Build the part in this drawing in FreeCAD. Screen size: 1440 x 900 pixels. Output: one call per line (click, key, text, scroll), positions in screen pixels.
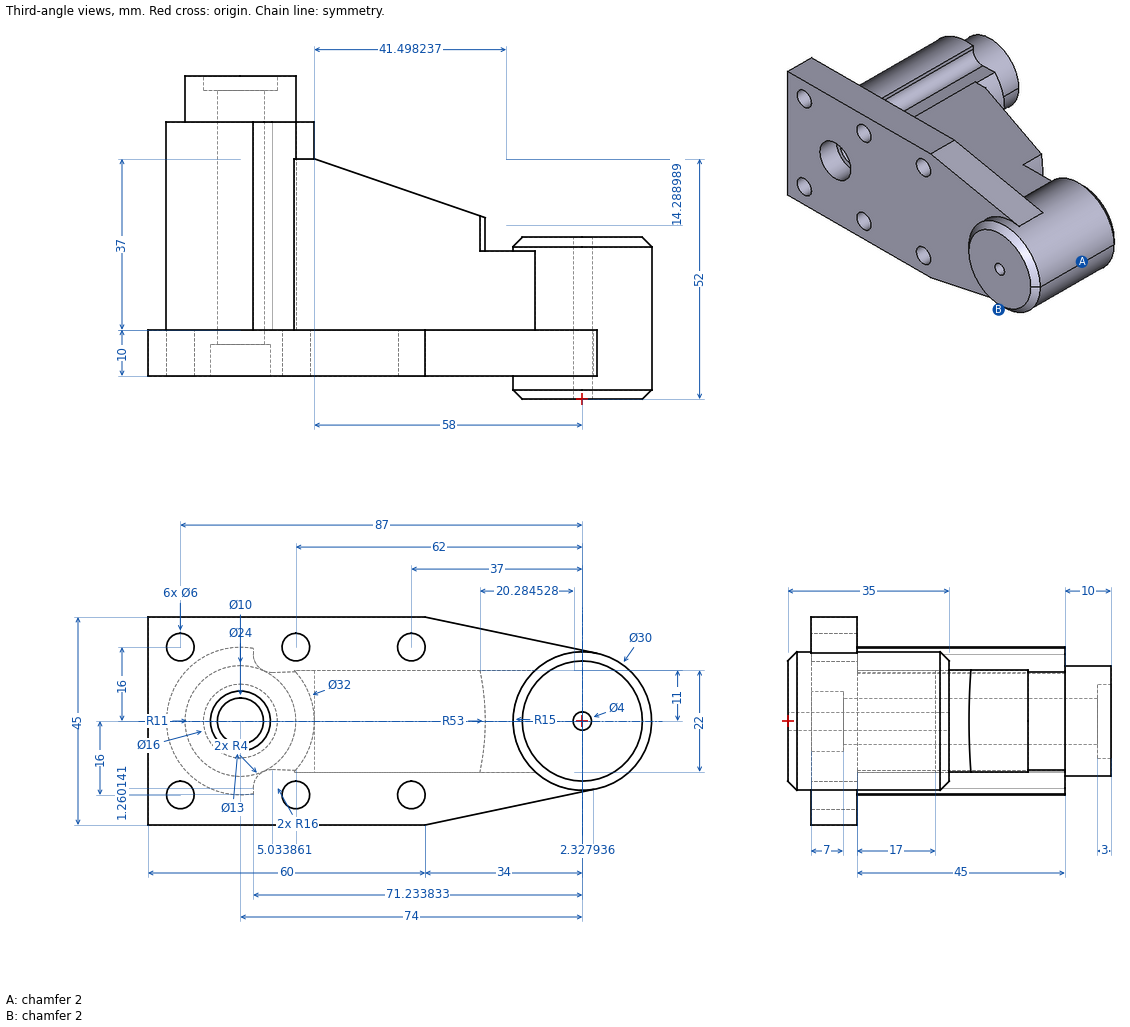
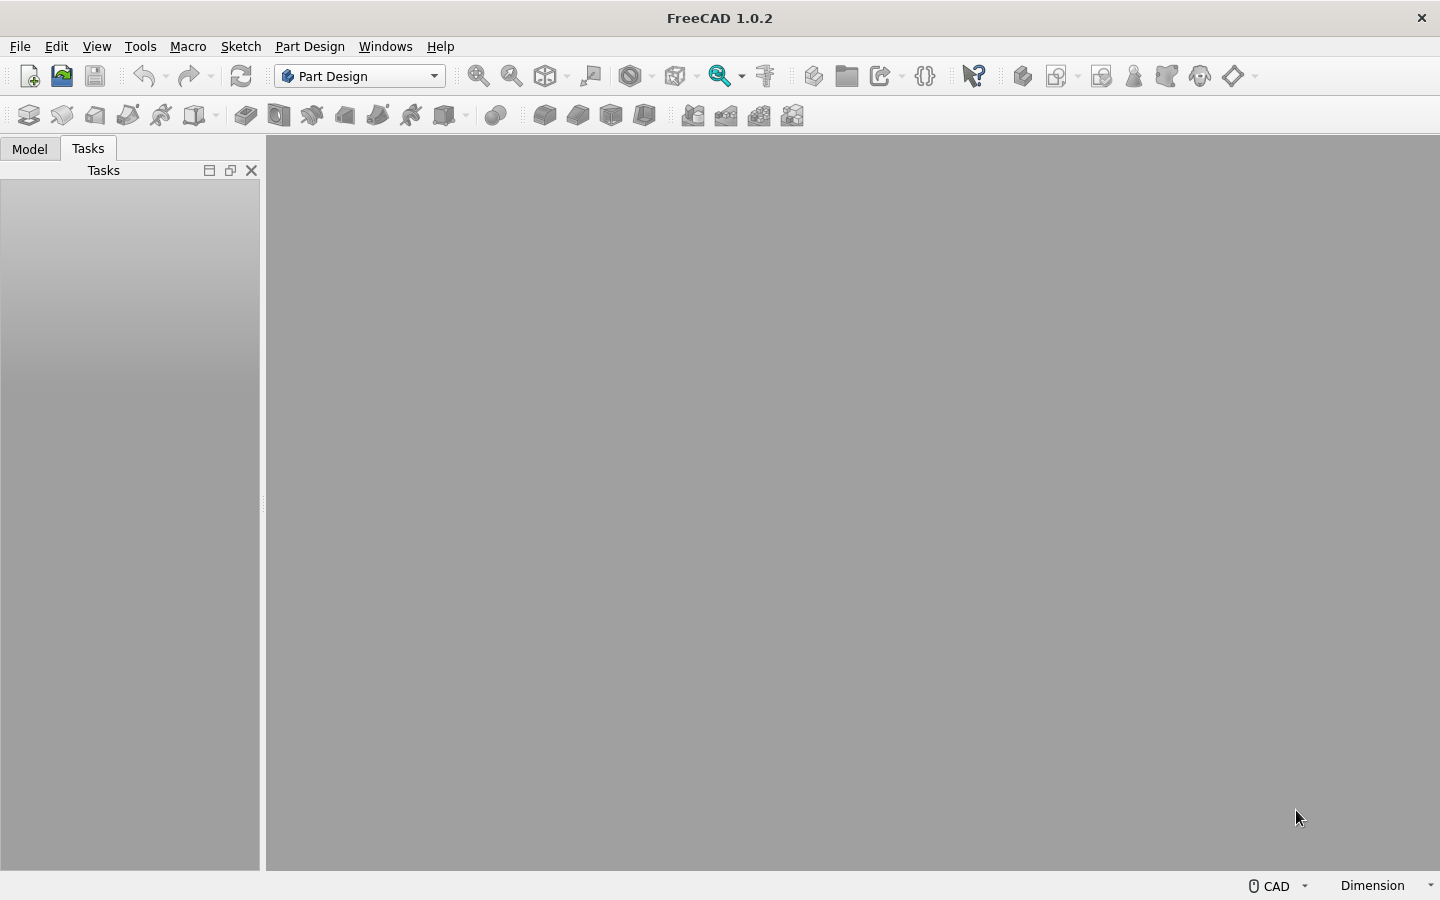
click(29, 76)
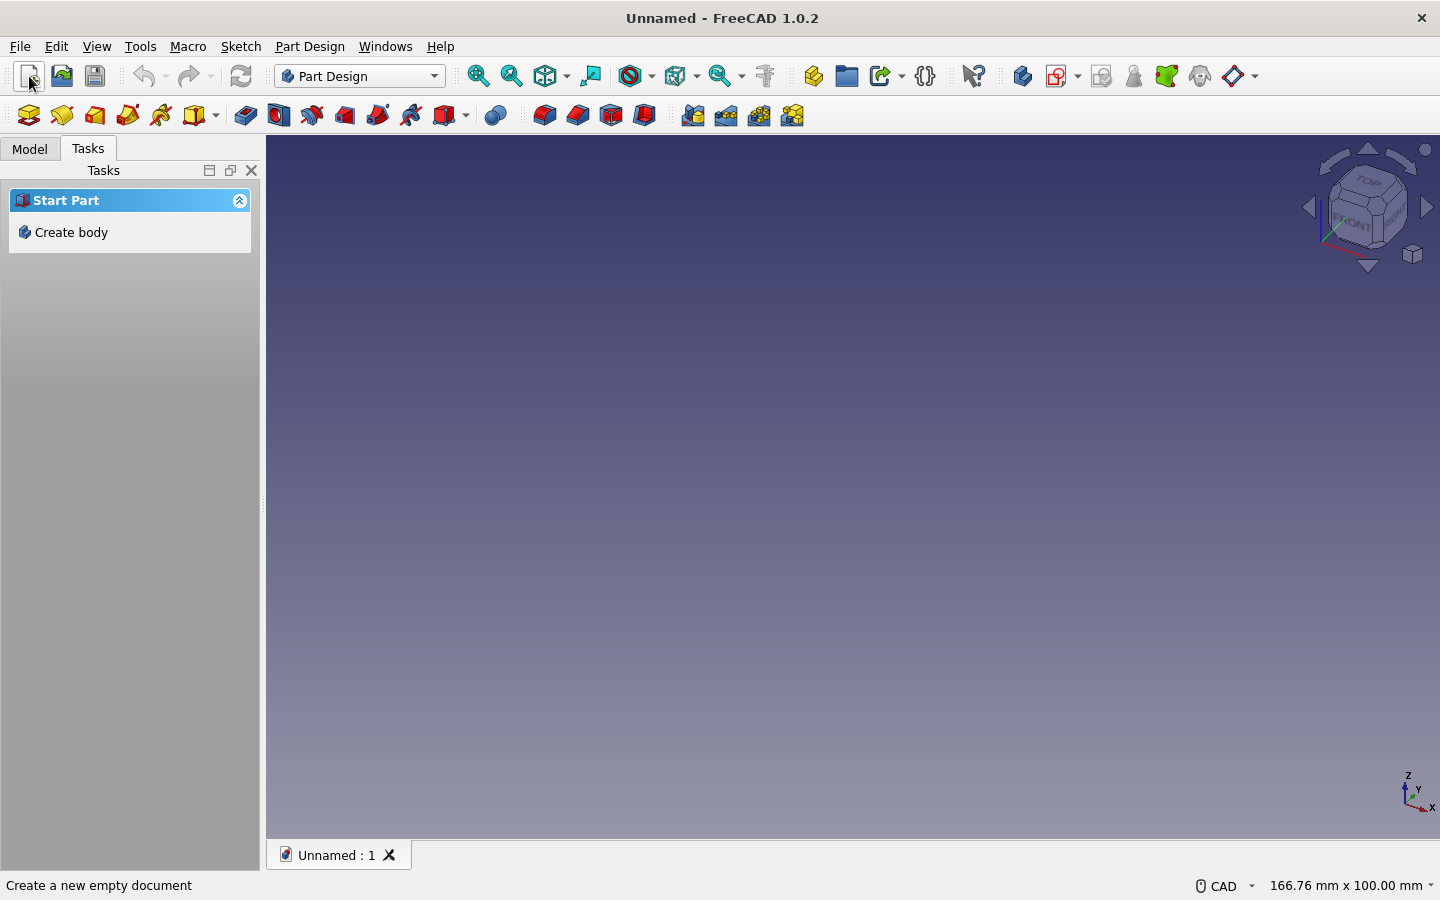
click(1056, 76)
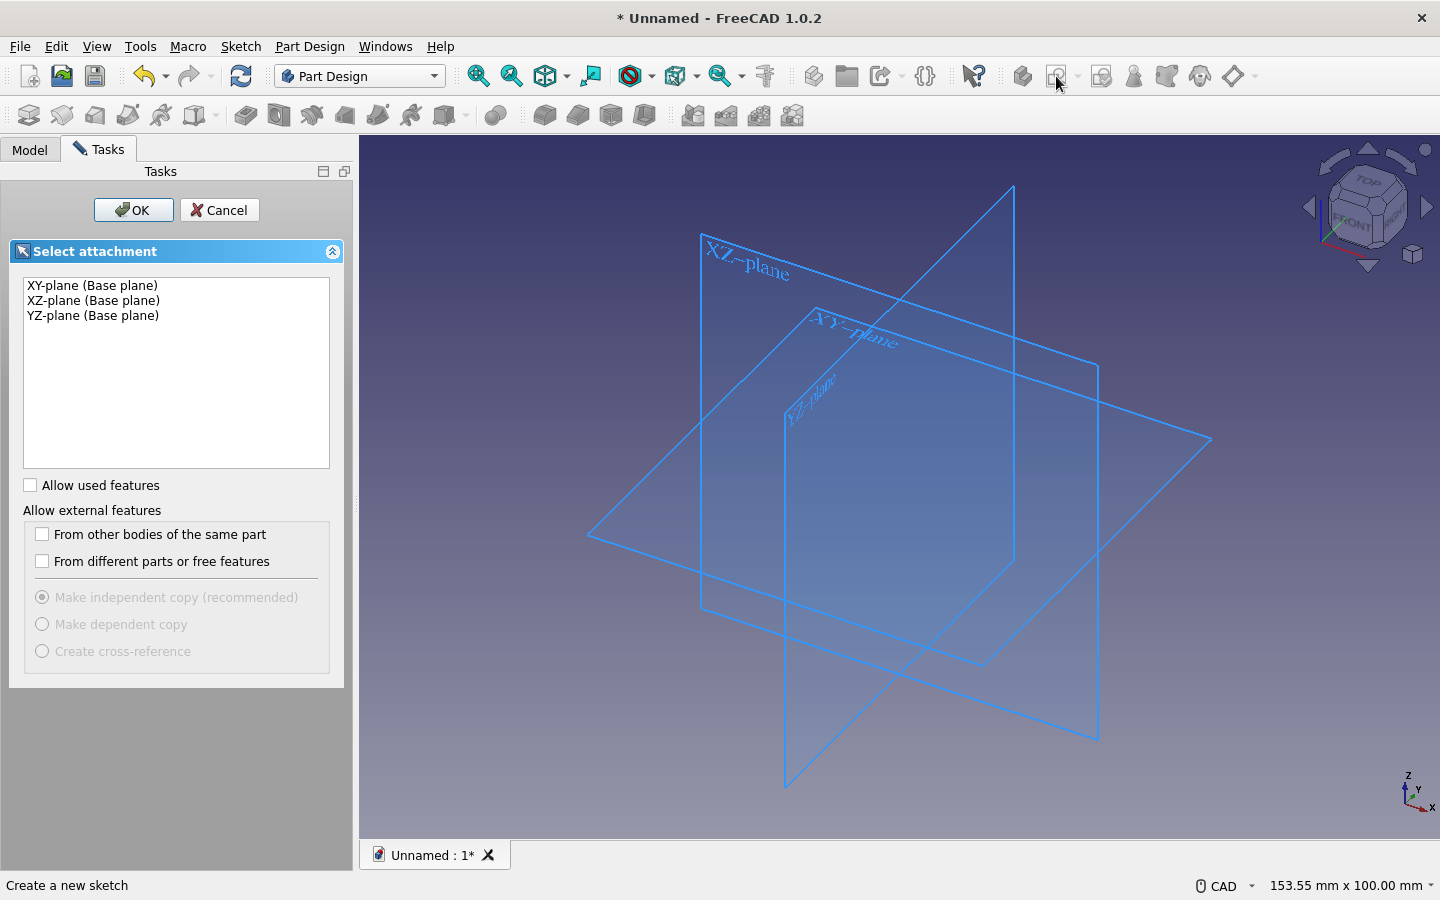
click(84, 300)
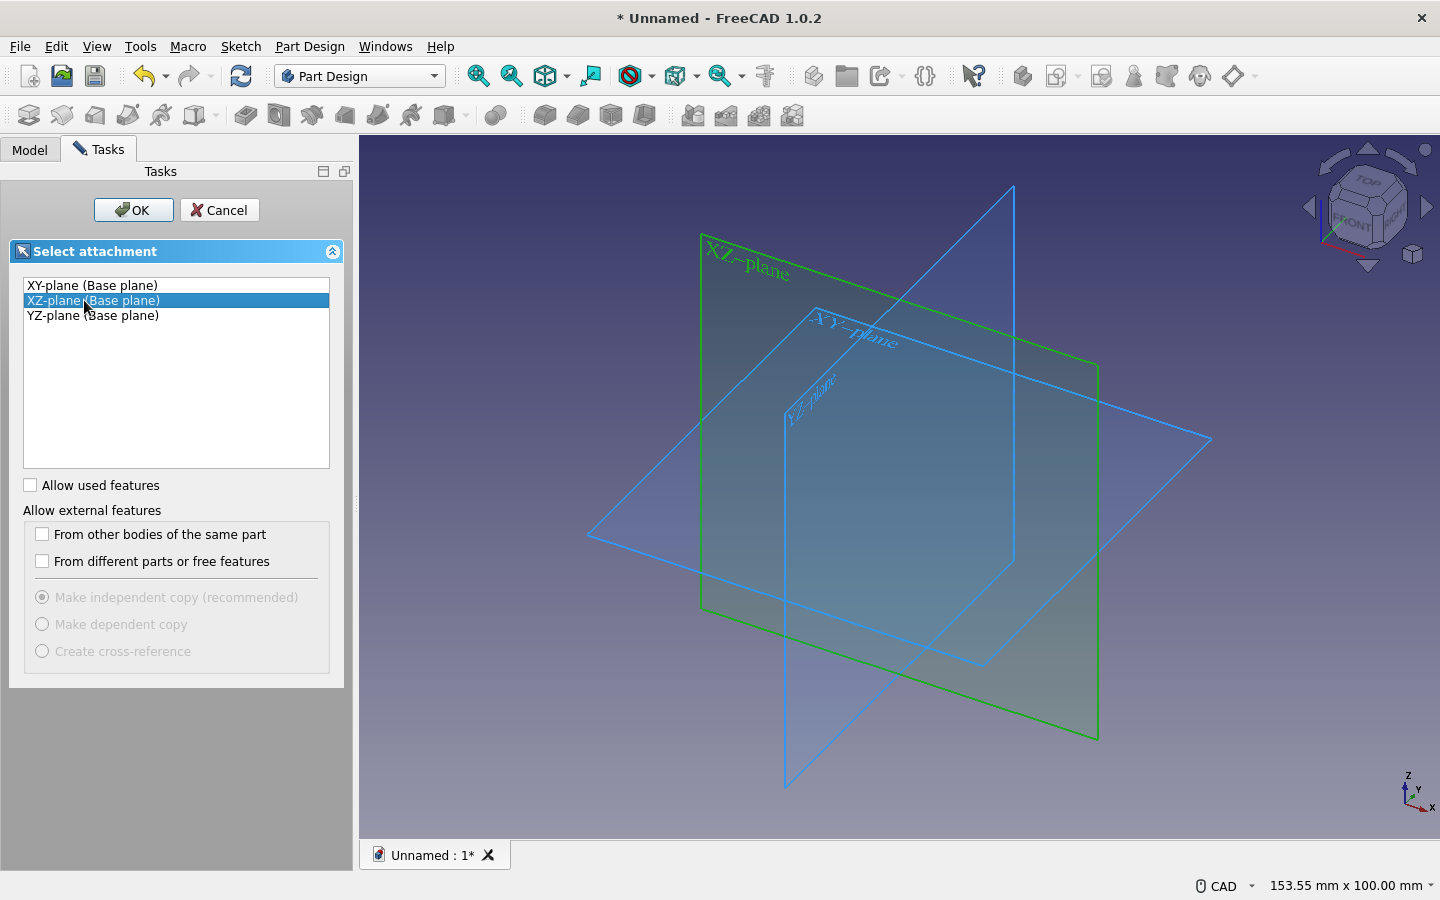
click(134, 210)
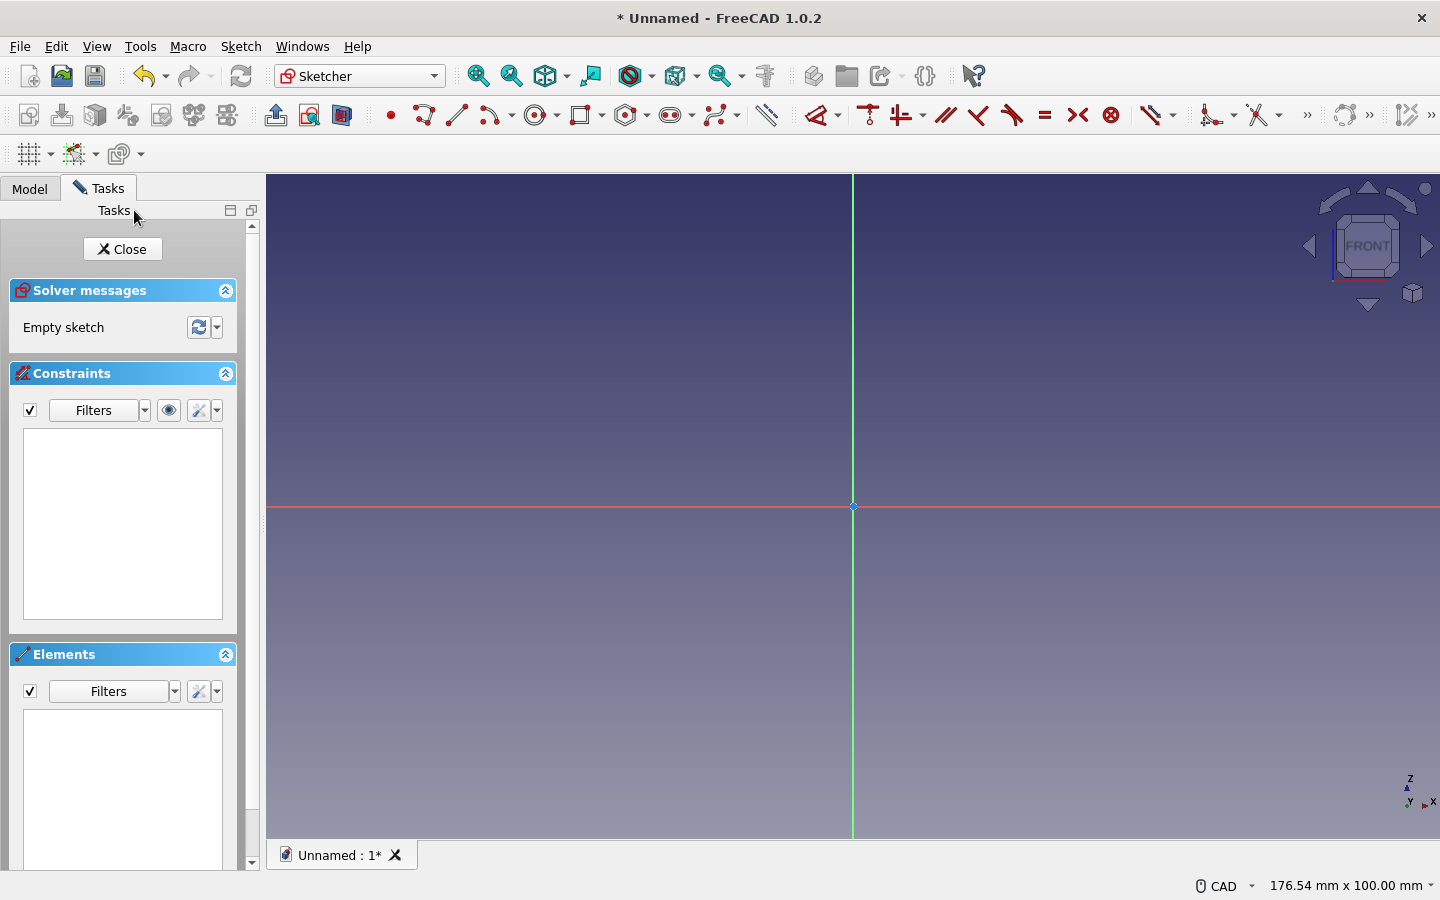
scroll(909, 506, up, 4)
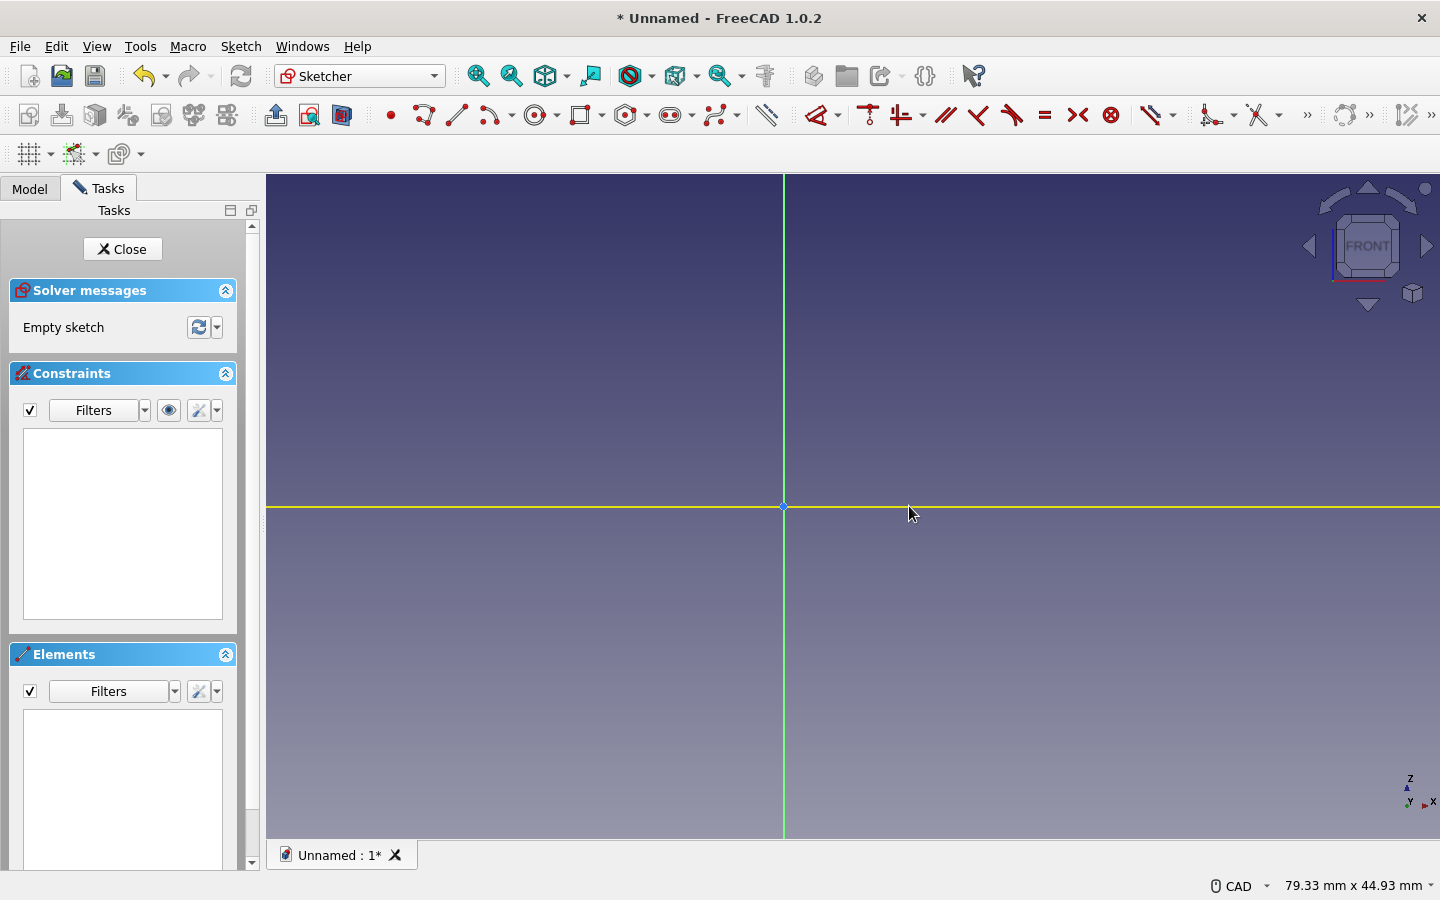
click(534, 116)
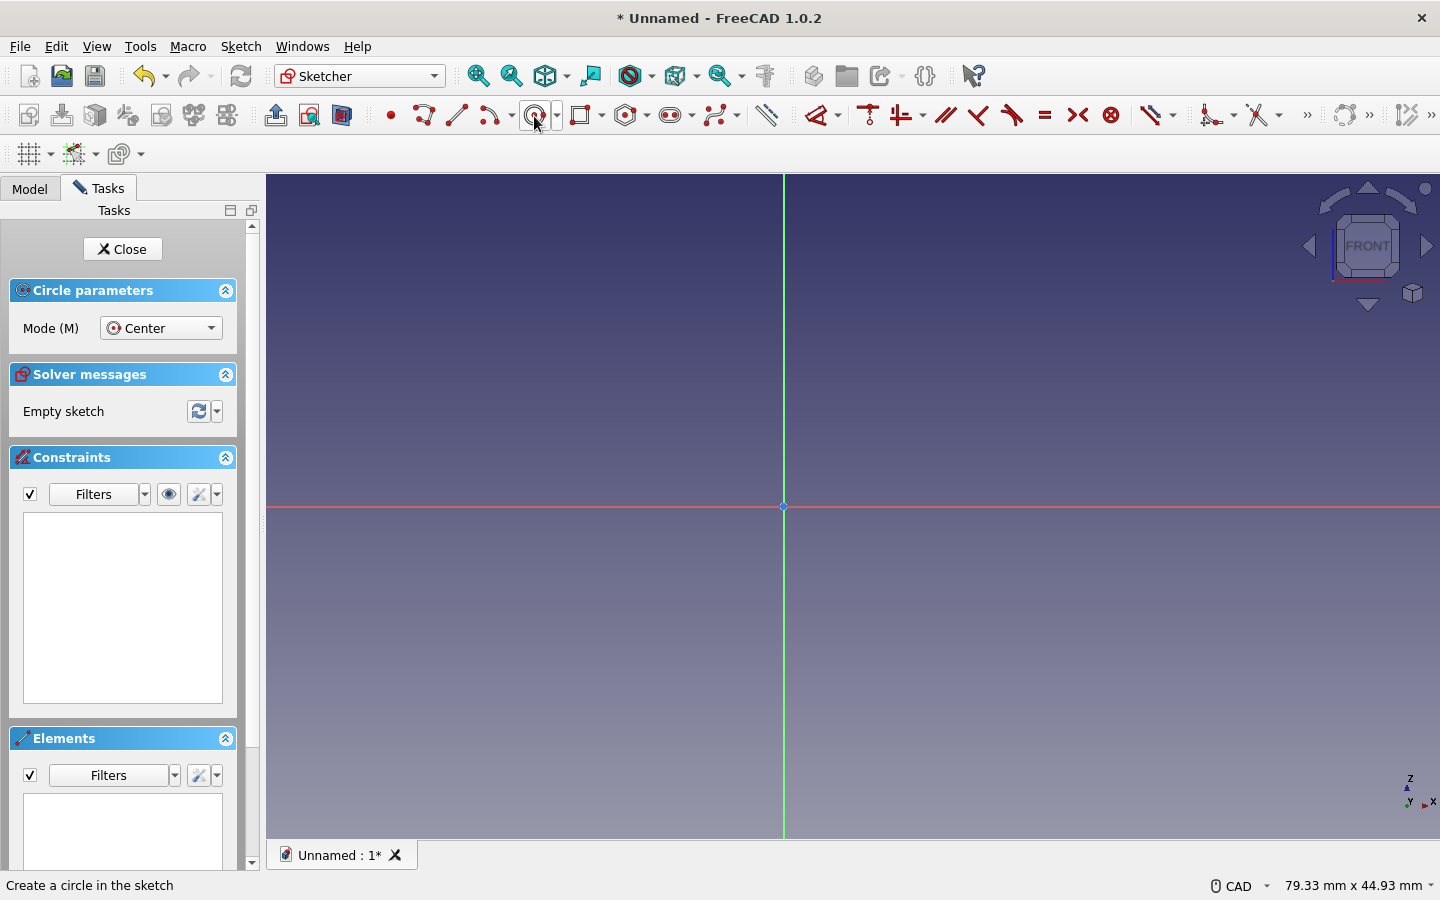
click(784, 506)
click(941, 350)
key(Escape)